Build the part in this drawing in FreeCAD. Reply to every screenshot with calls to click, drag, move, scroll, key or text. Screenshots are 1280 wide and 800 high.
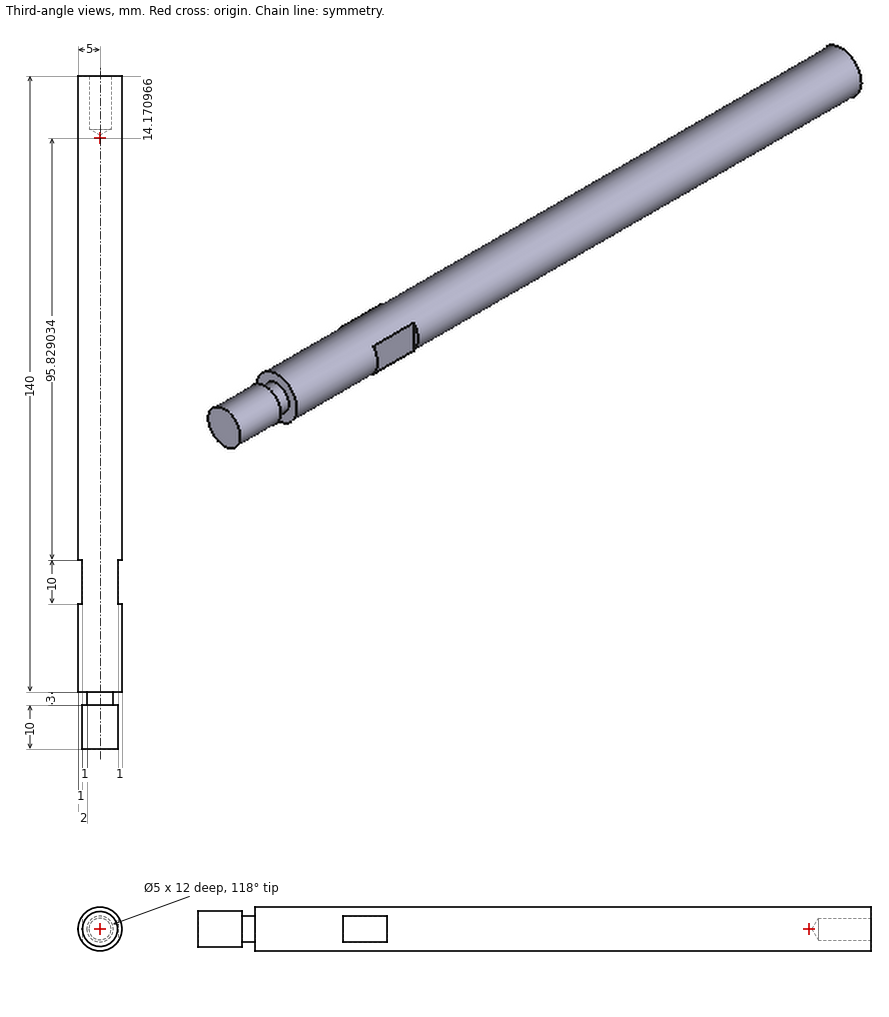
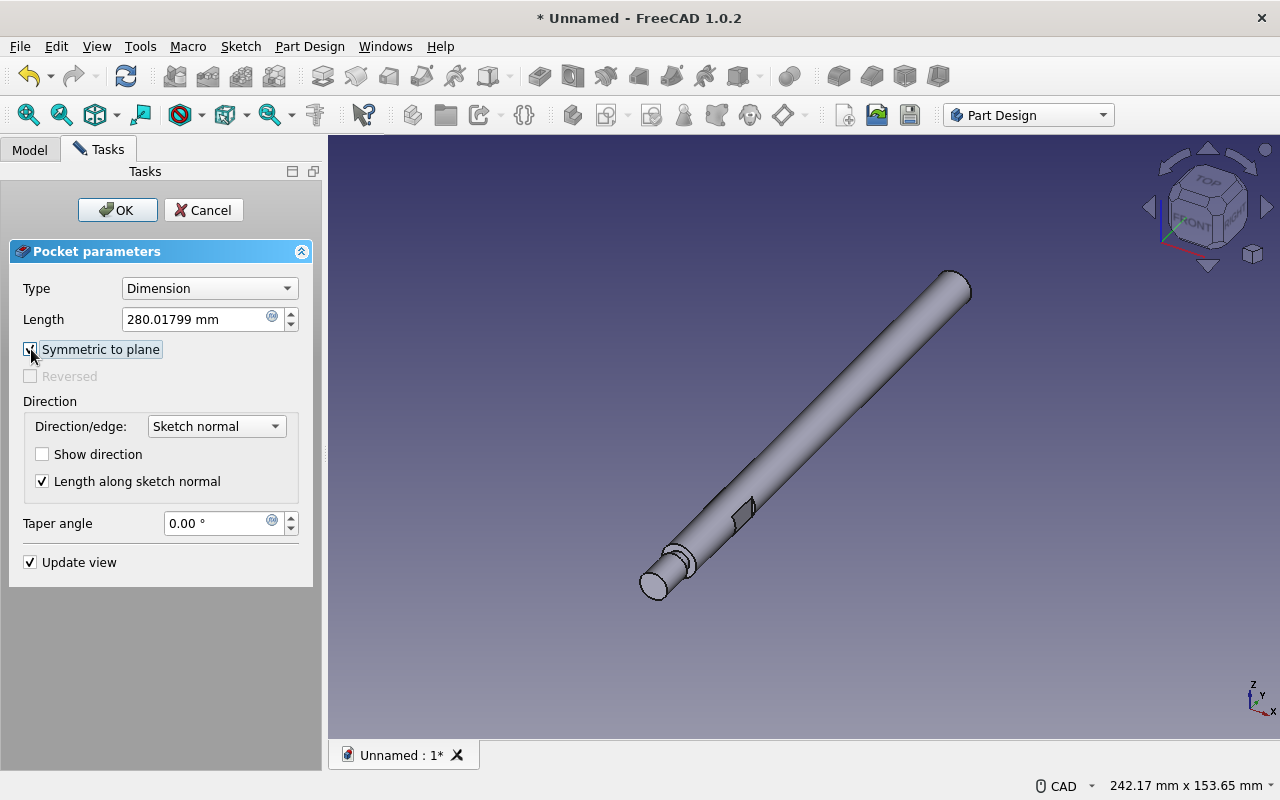
click(118, 210)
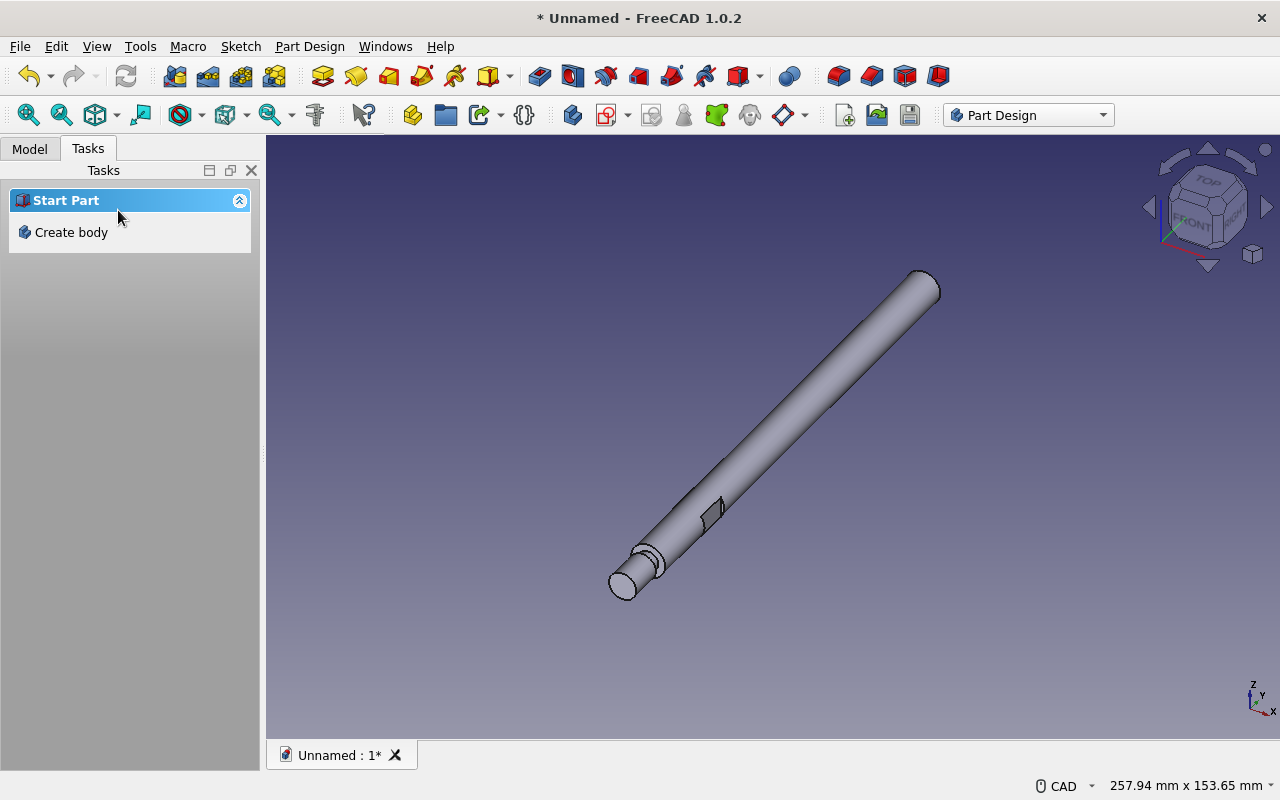
key(4)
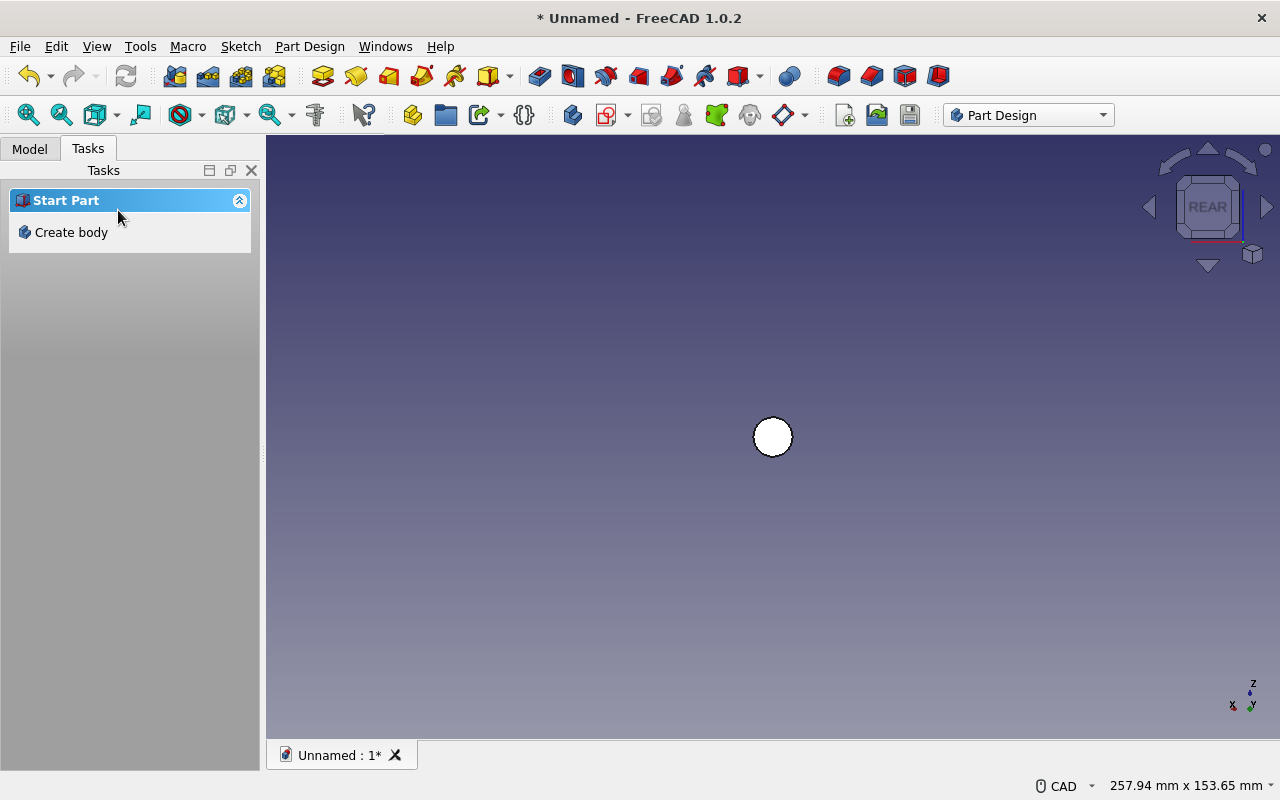
click(29, 116)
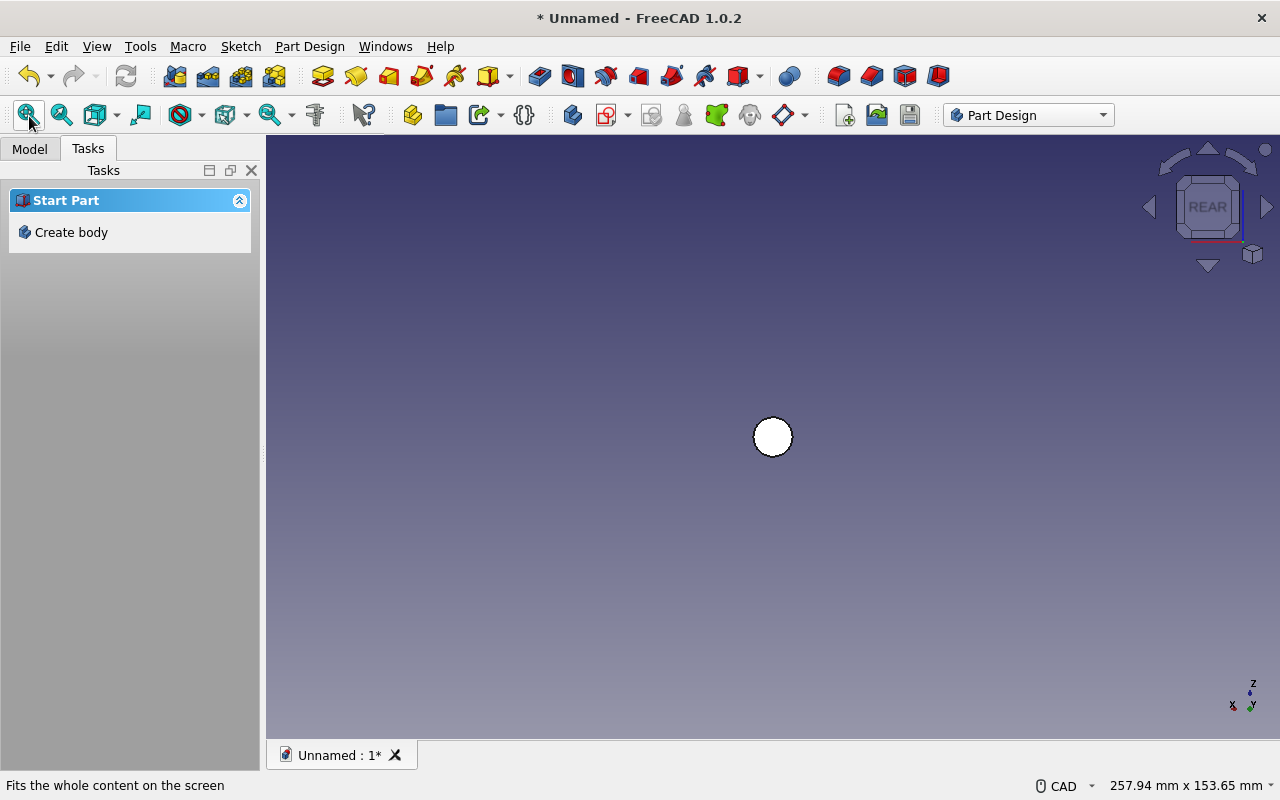
click(773, 436)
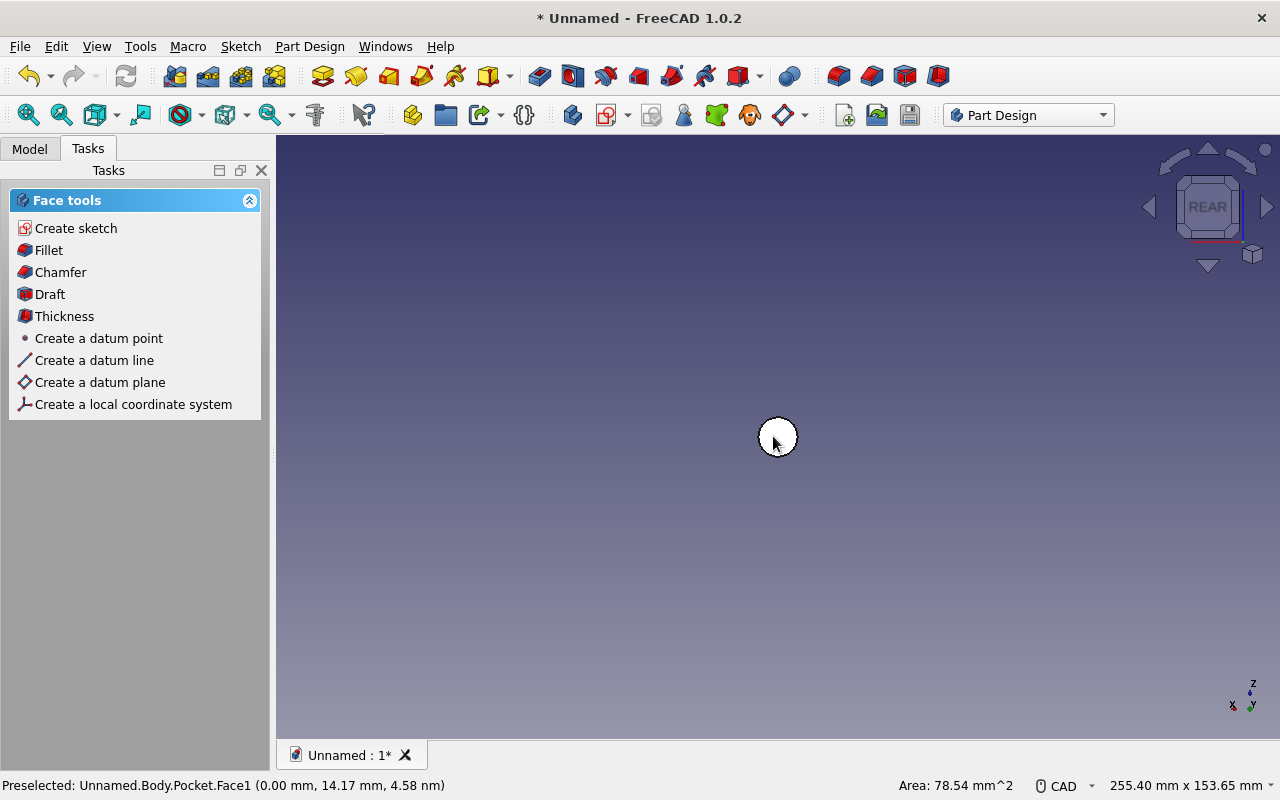
click(606, 116)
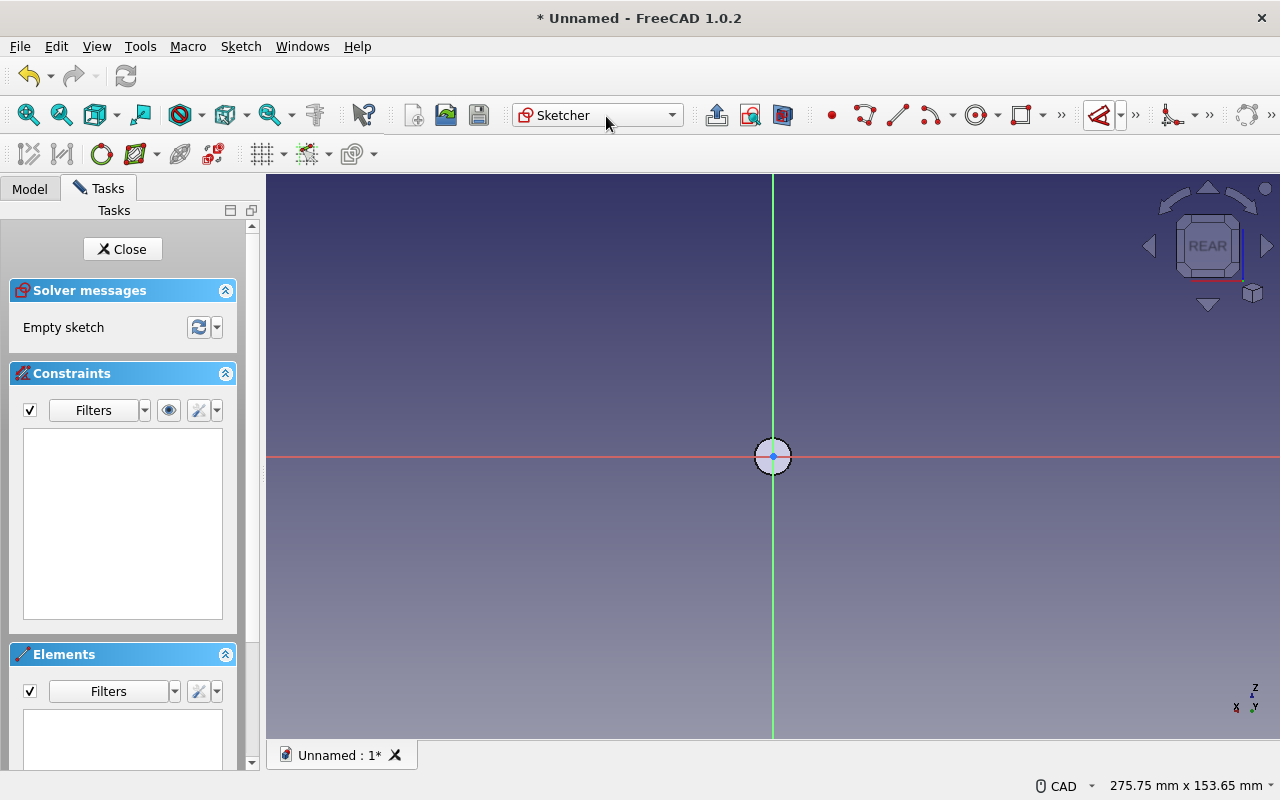
scroll(777, 457, up, 15)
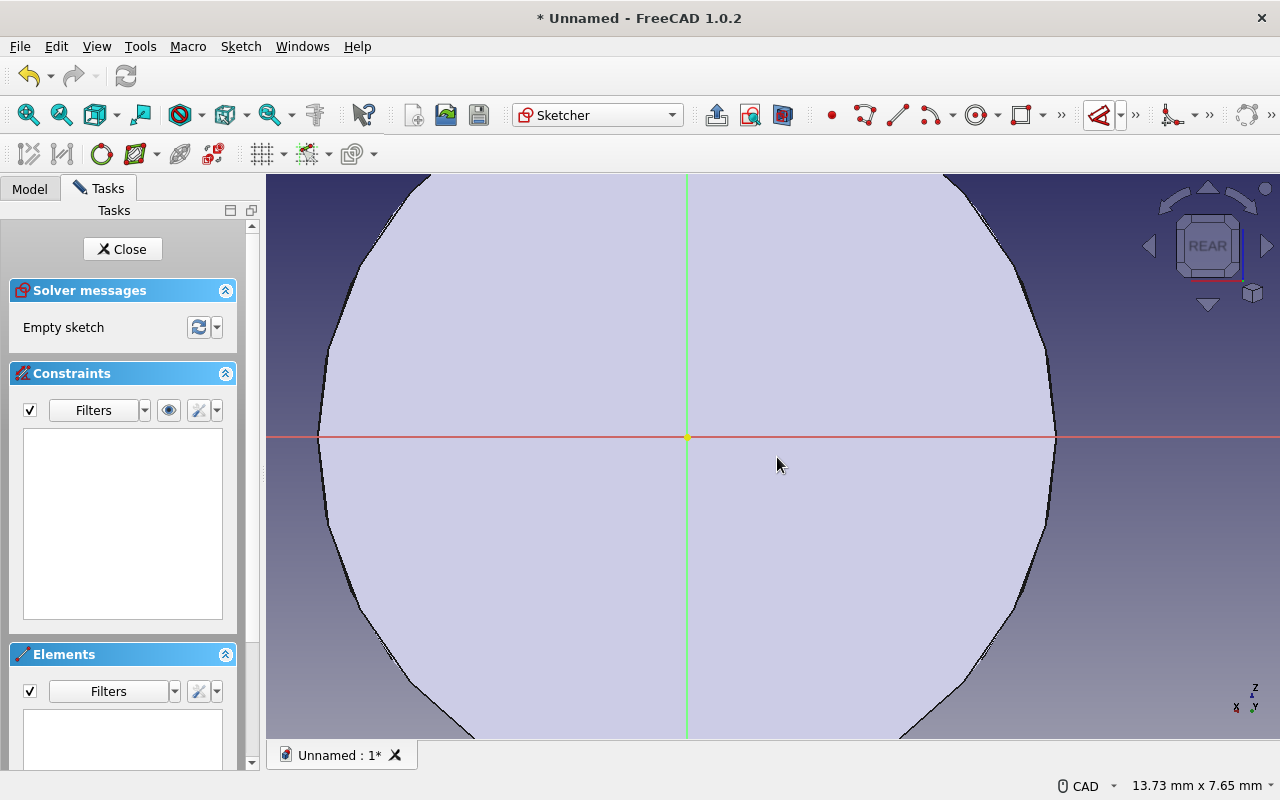
click(976, 116)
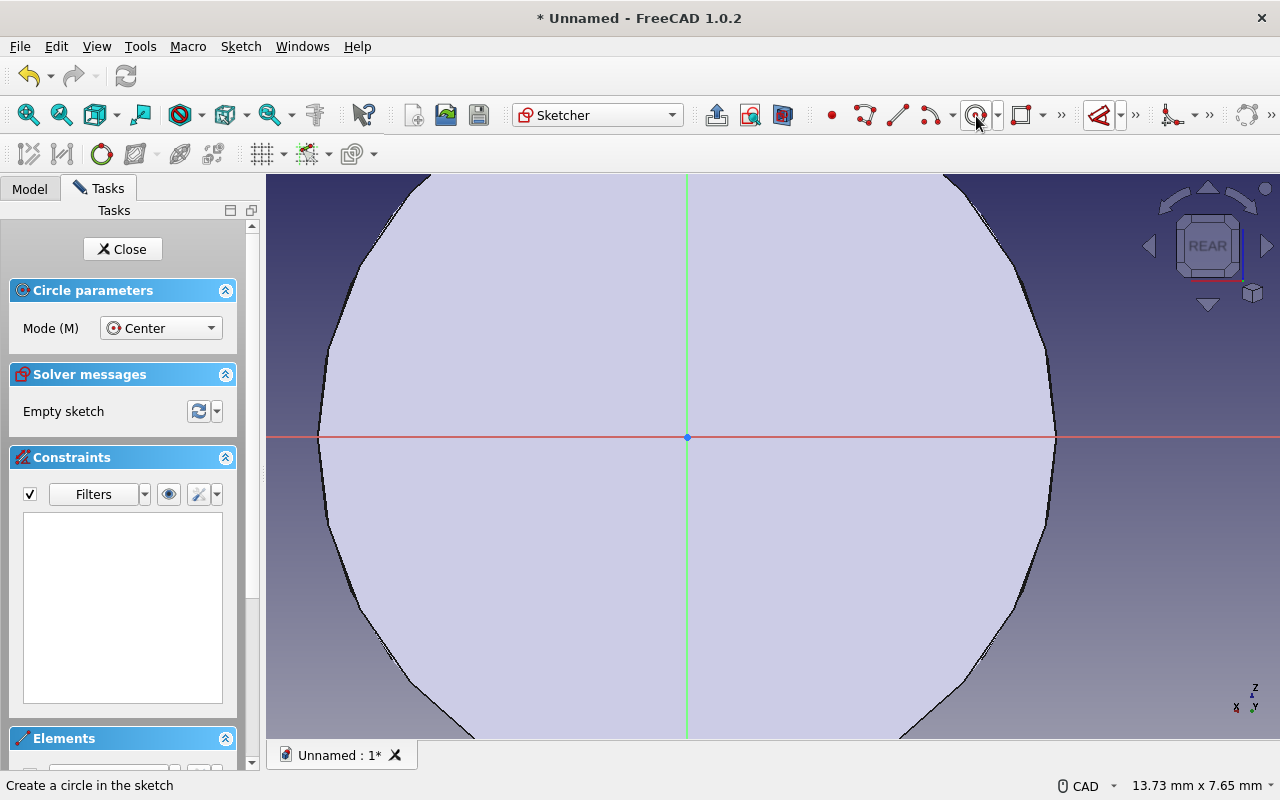
click(687, 437)
move(818, 307)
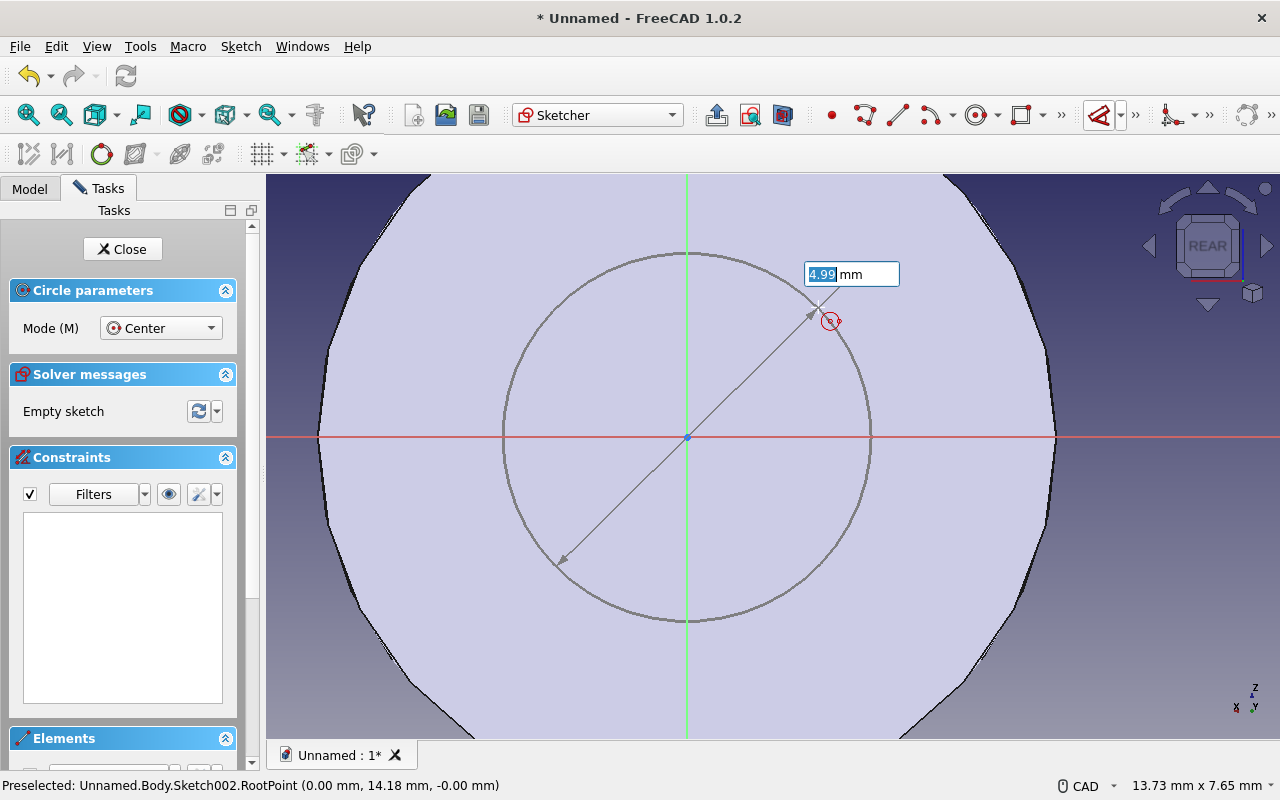
text(5)
key(Return)
key(Escape)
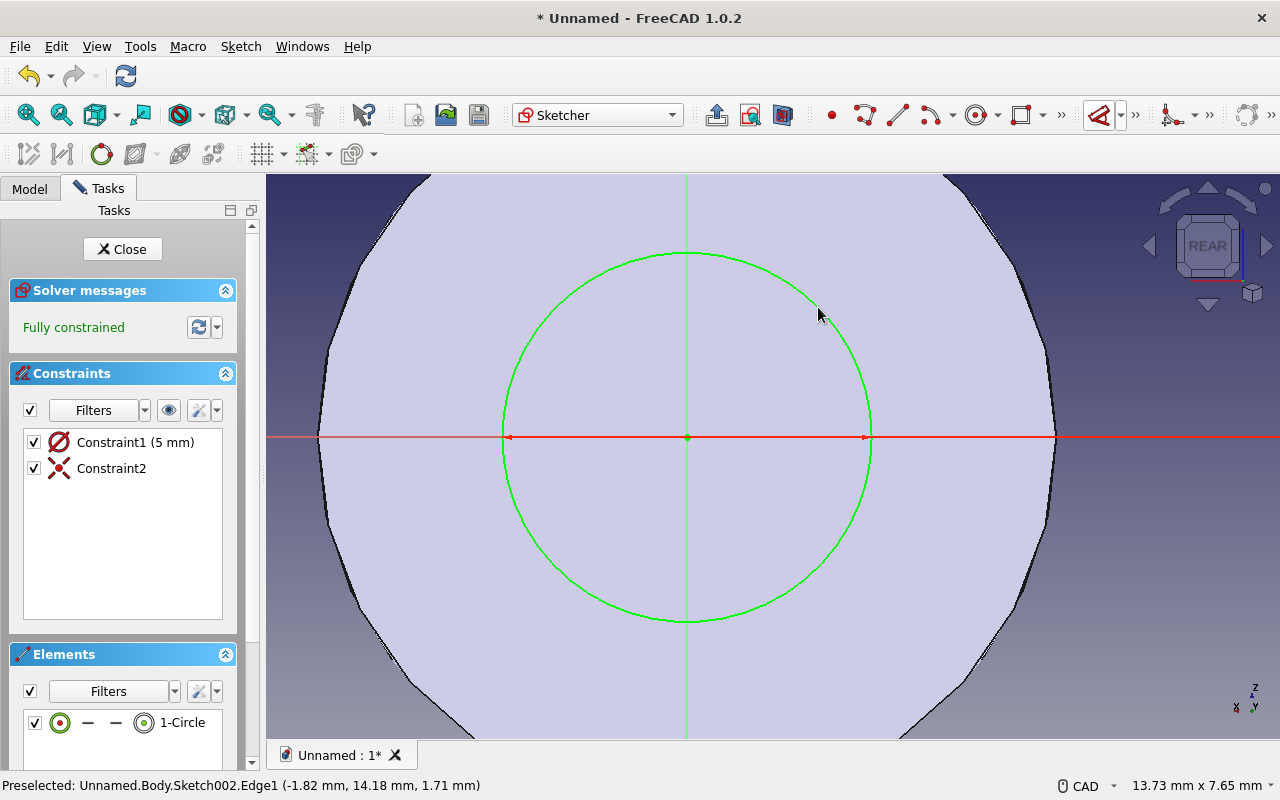
click(123, 249)